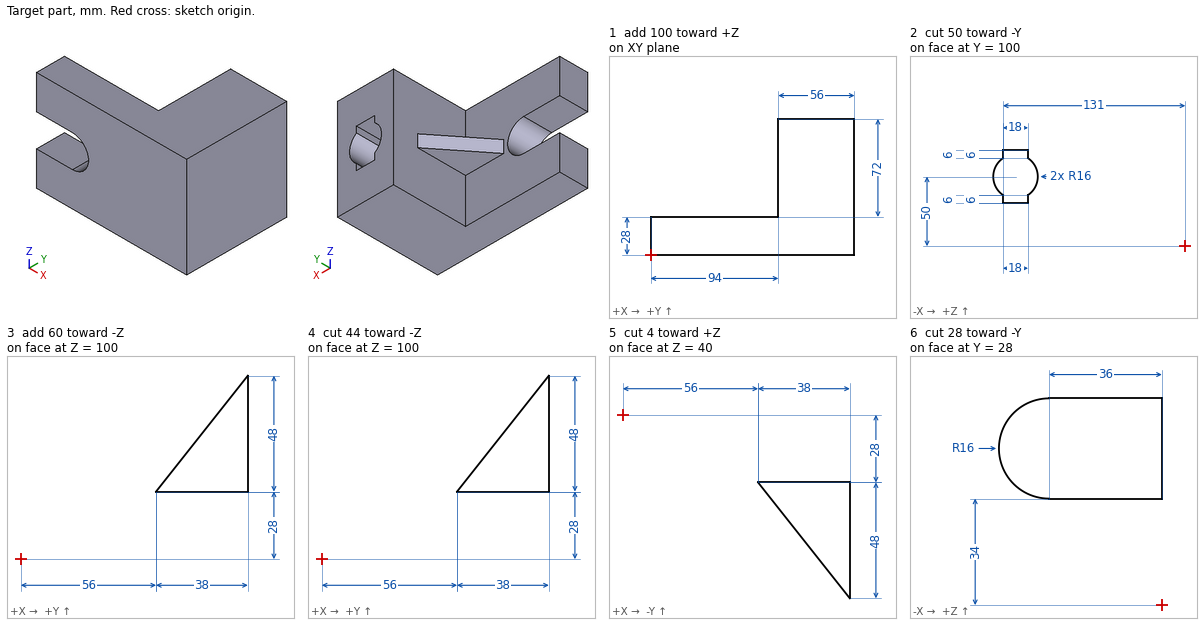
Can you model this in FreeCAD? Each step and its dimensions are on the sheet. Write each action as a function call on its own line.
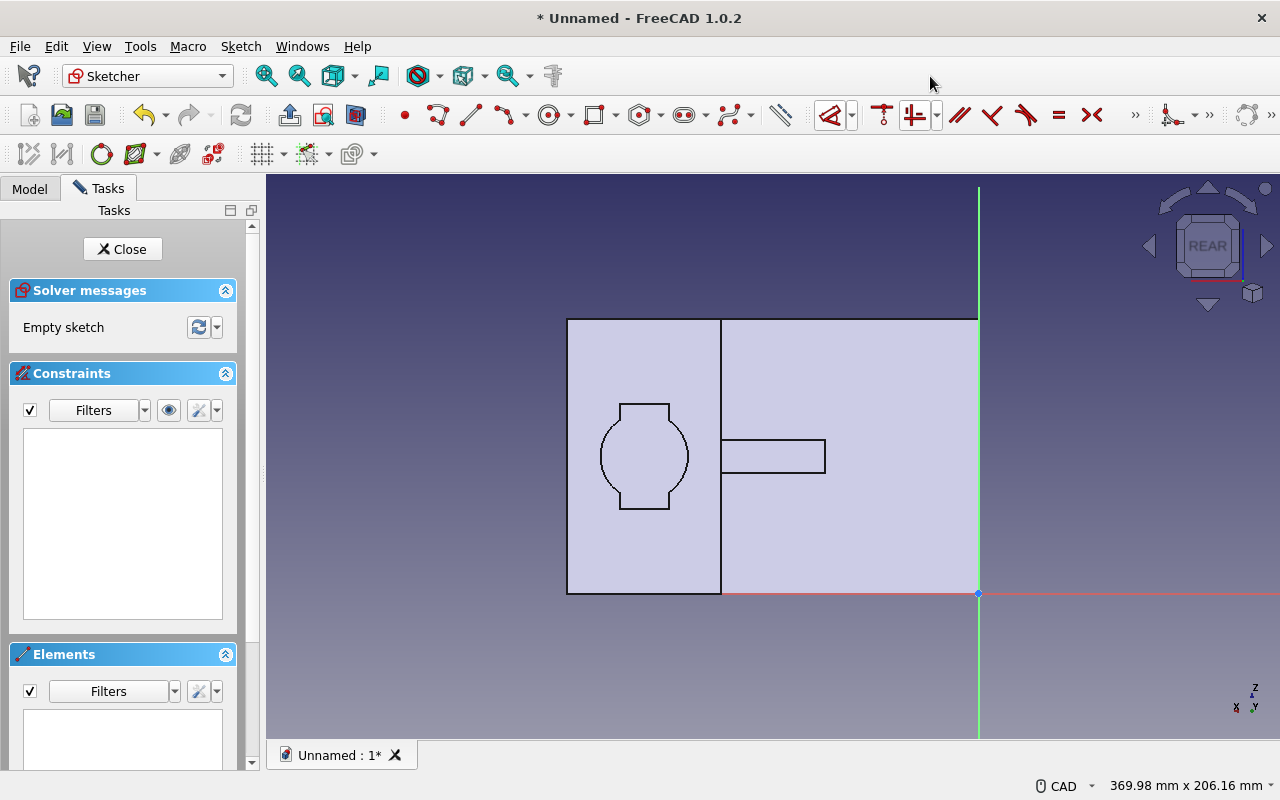
scroll(1115, 560, up, 3)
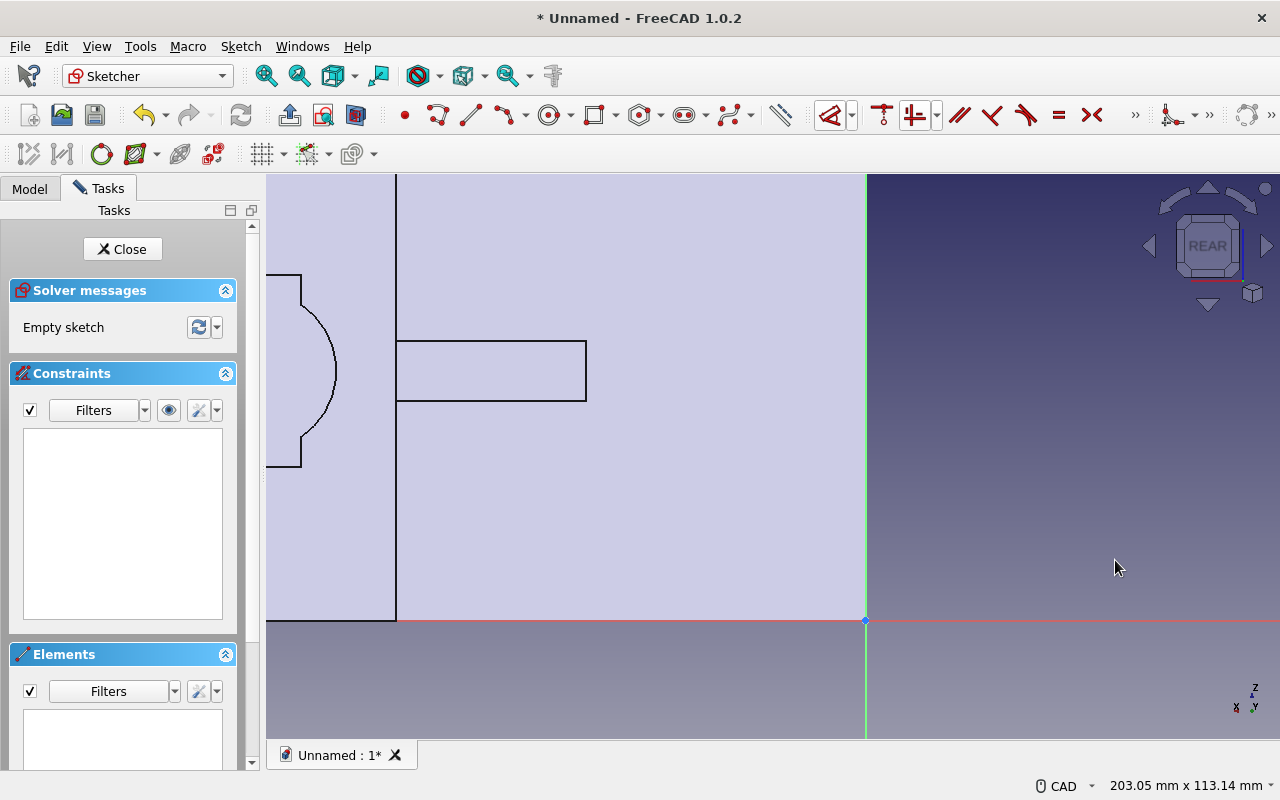
click(438, 116)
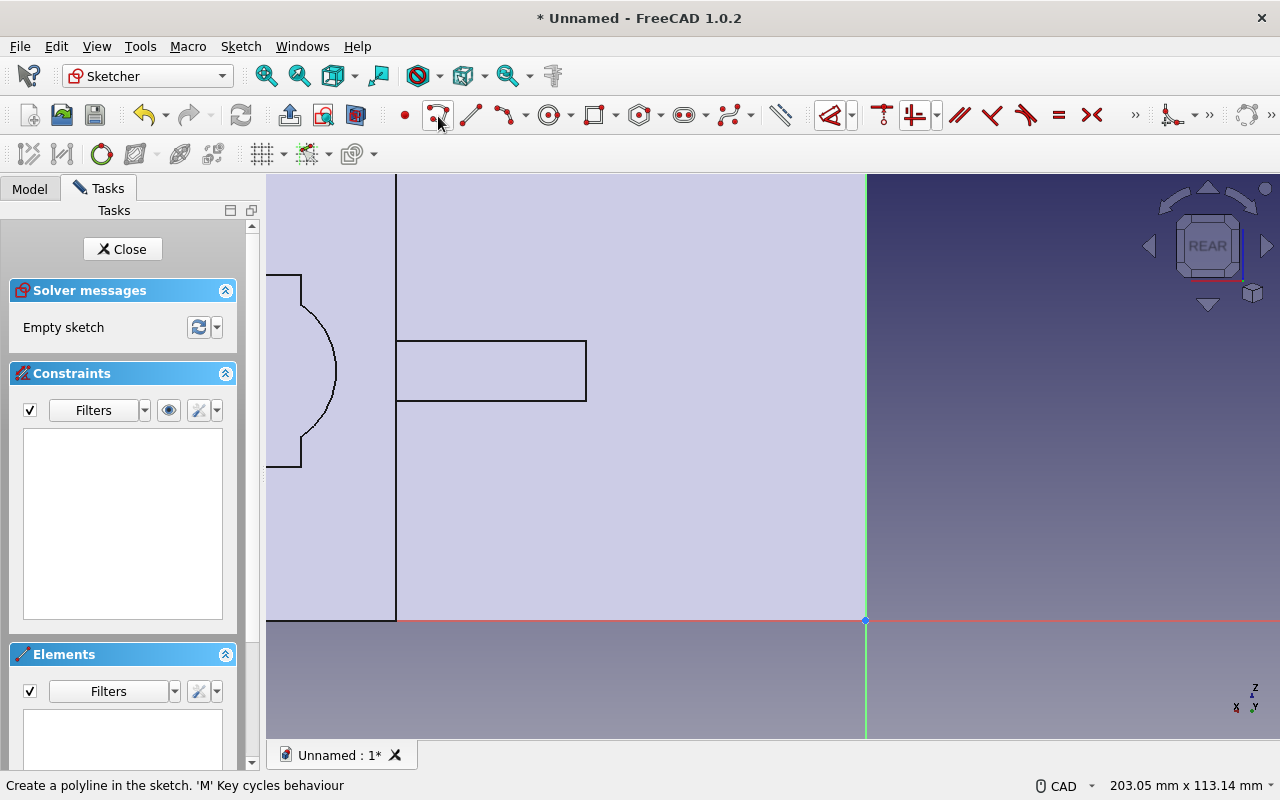
click(686, 451)
click(866, 451)
click(857, 291)
click(686, 291)
right_click(686, 291)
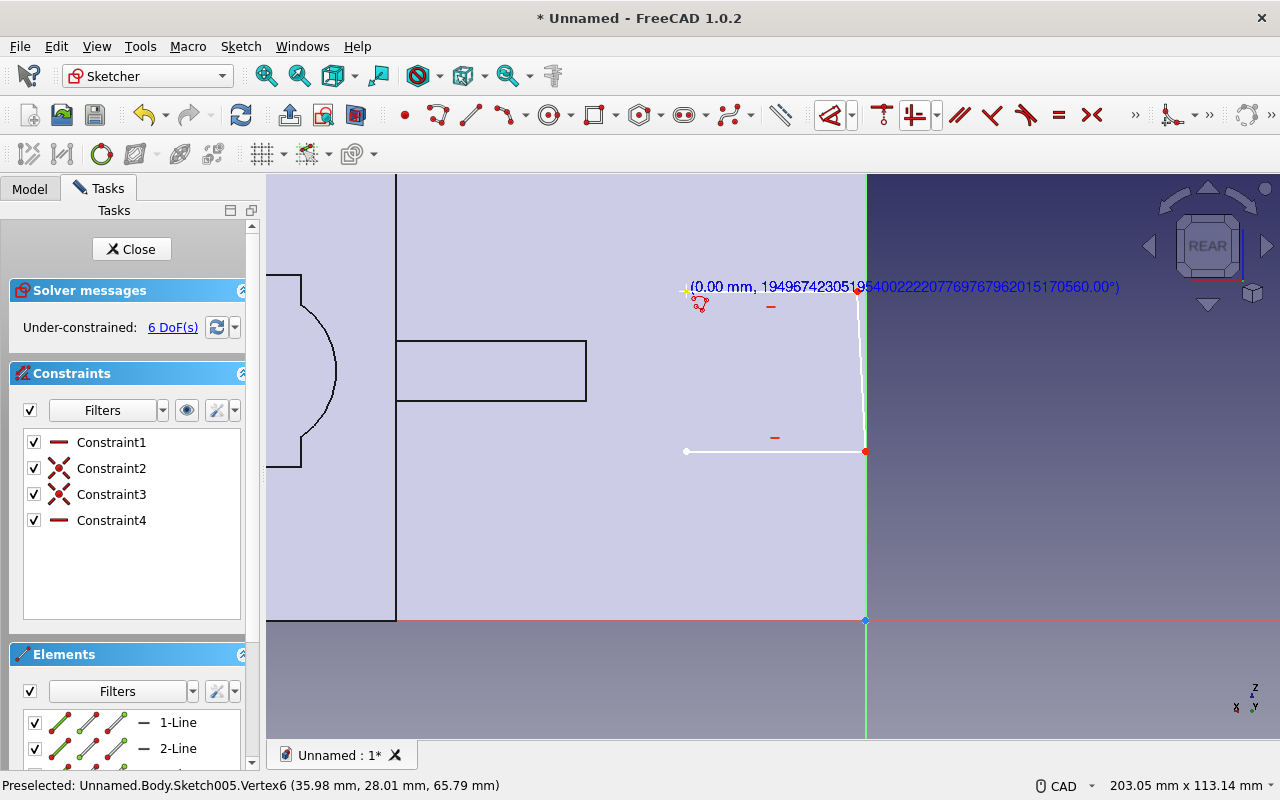
click(504, 116)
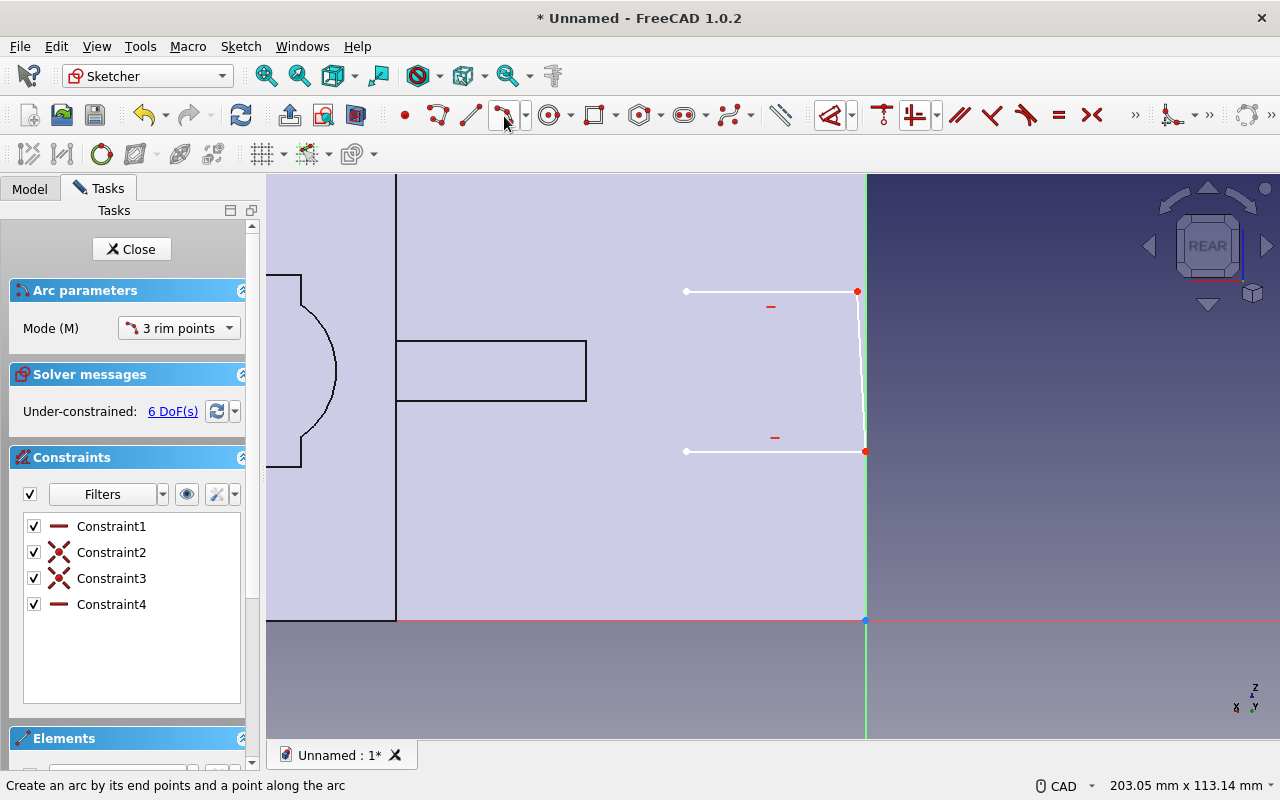
click(686, 292)
click(686, 452)
click(606, 371)
key(Escape)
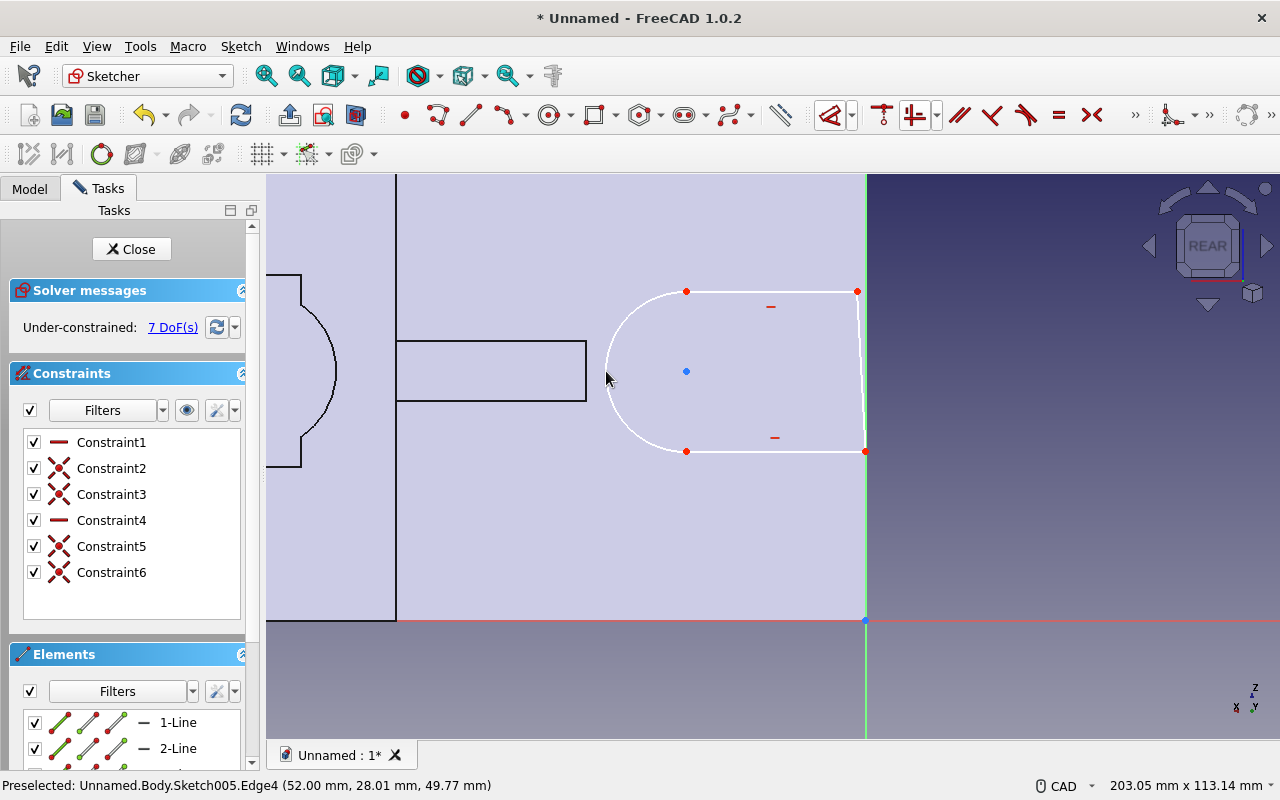
click(740, 452)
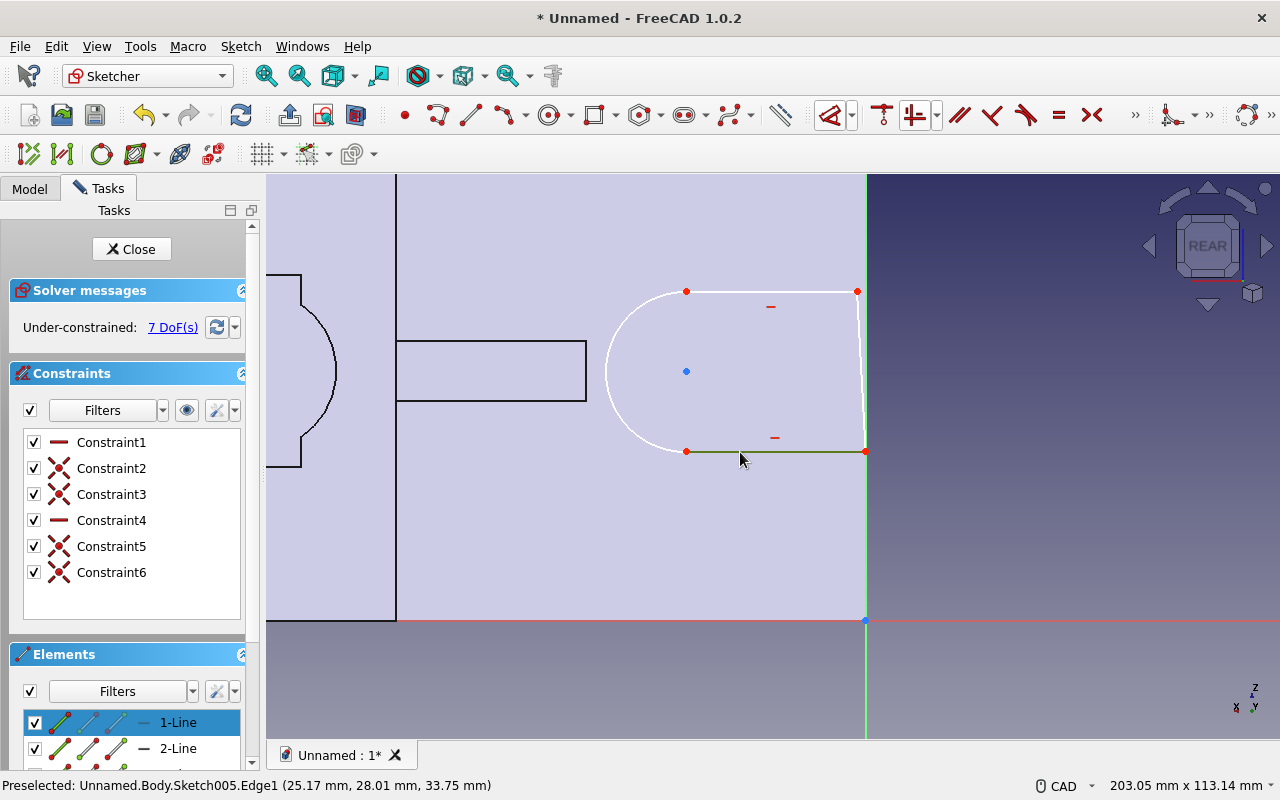
click(621, 325)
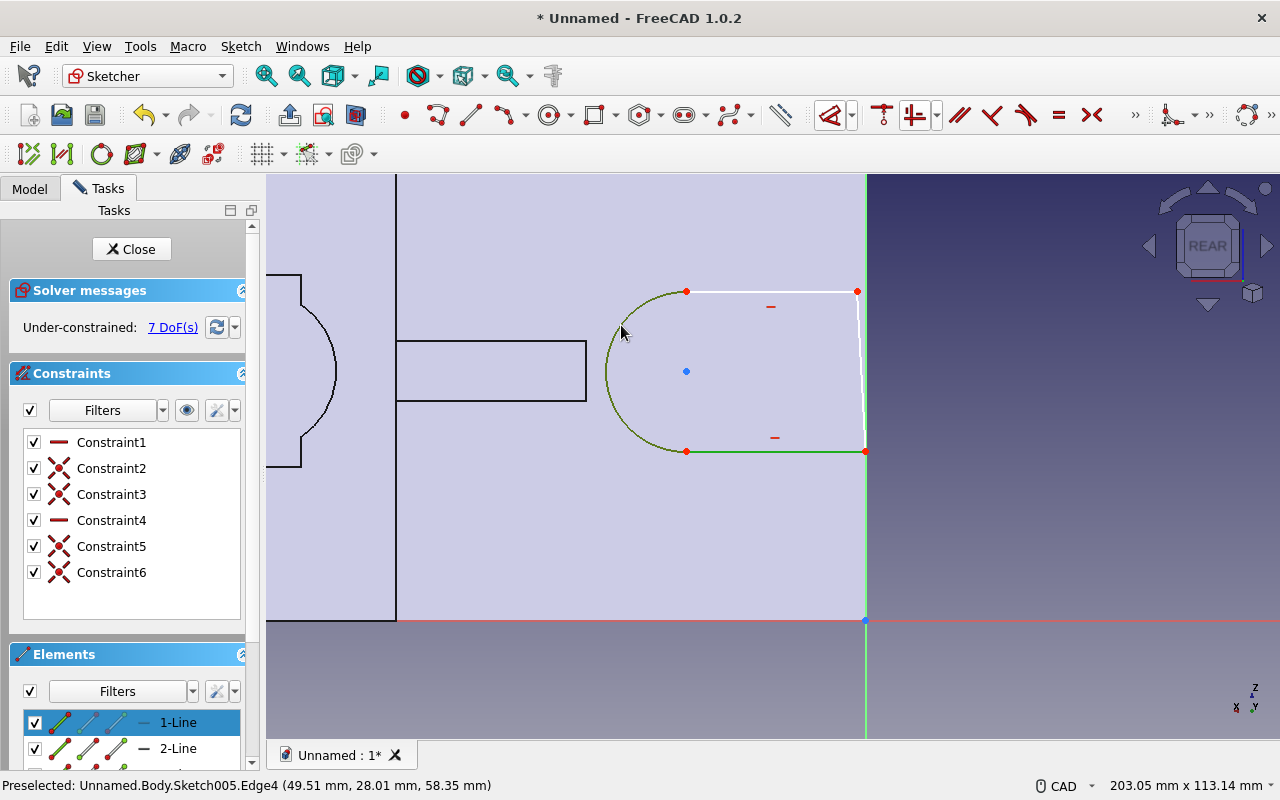
click(1026, 116)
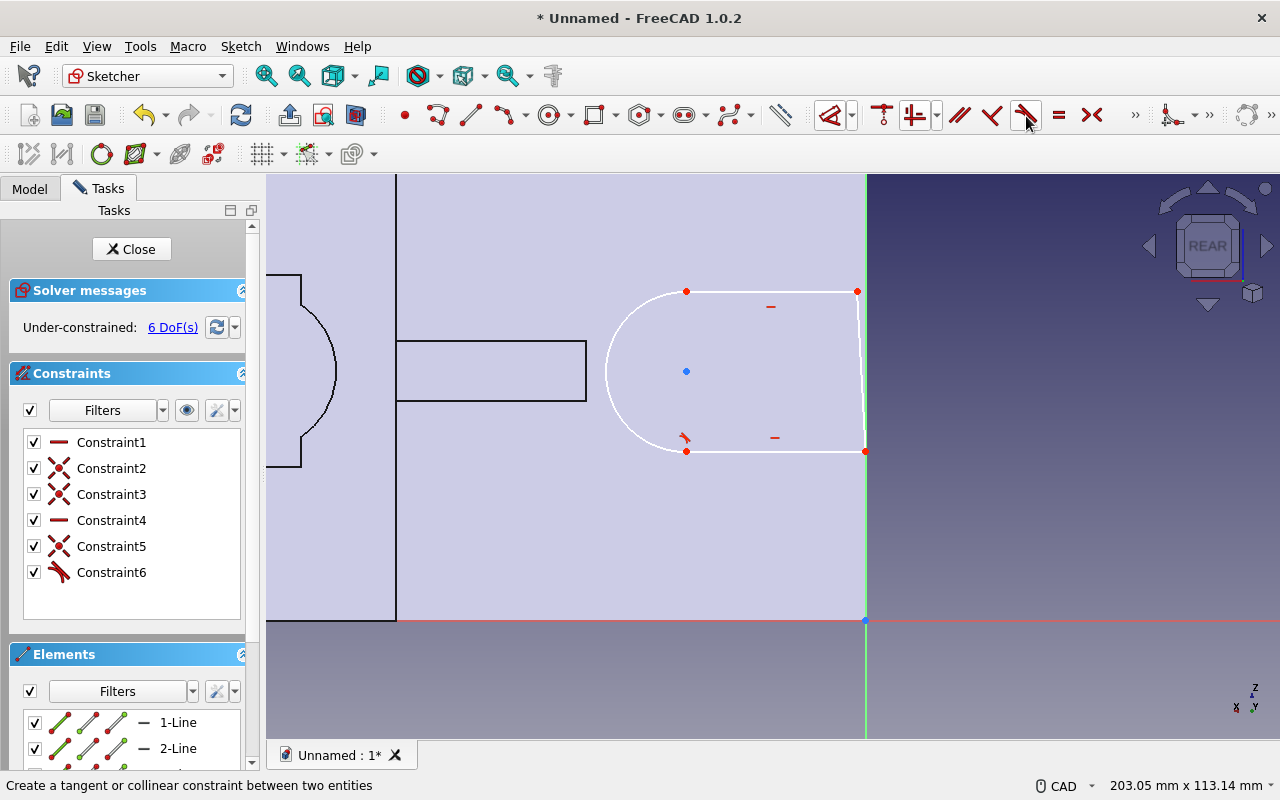
click(806, 292)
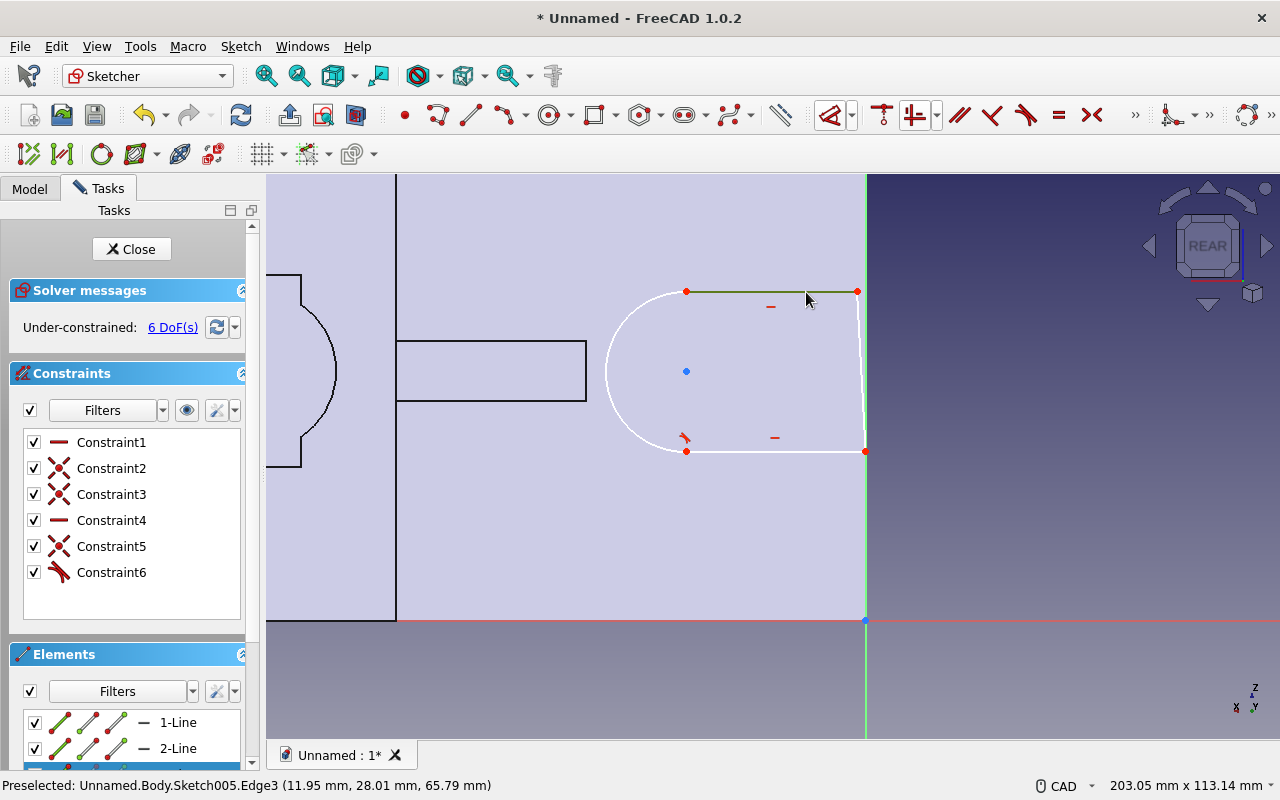
click(621, 325)